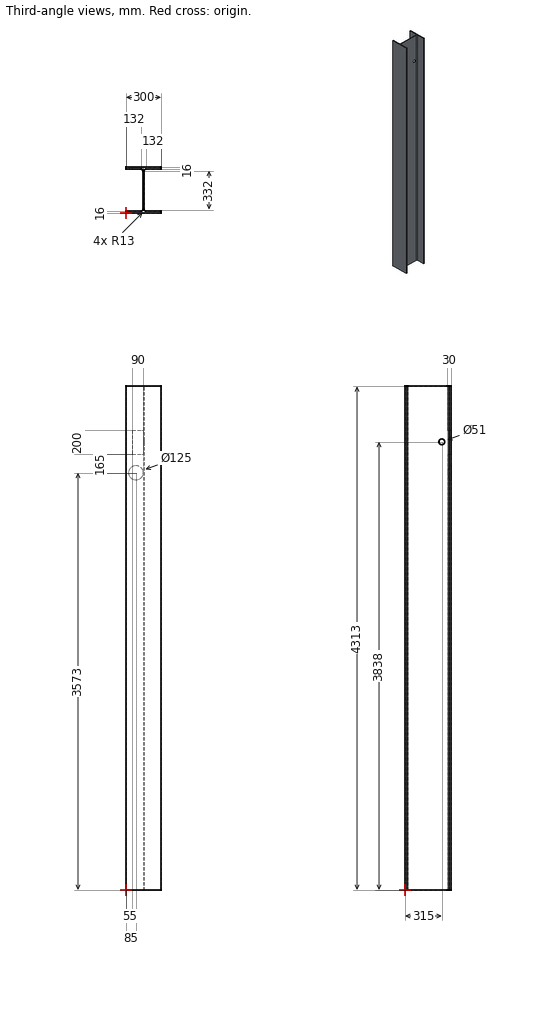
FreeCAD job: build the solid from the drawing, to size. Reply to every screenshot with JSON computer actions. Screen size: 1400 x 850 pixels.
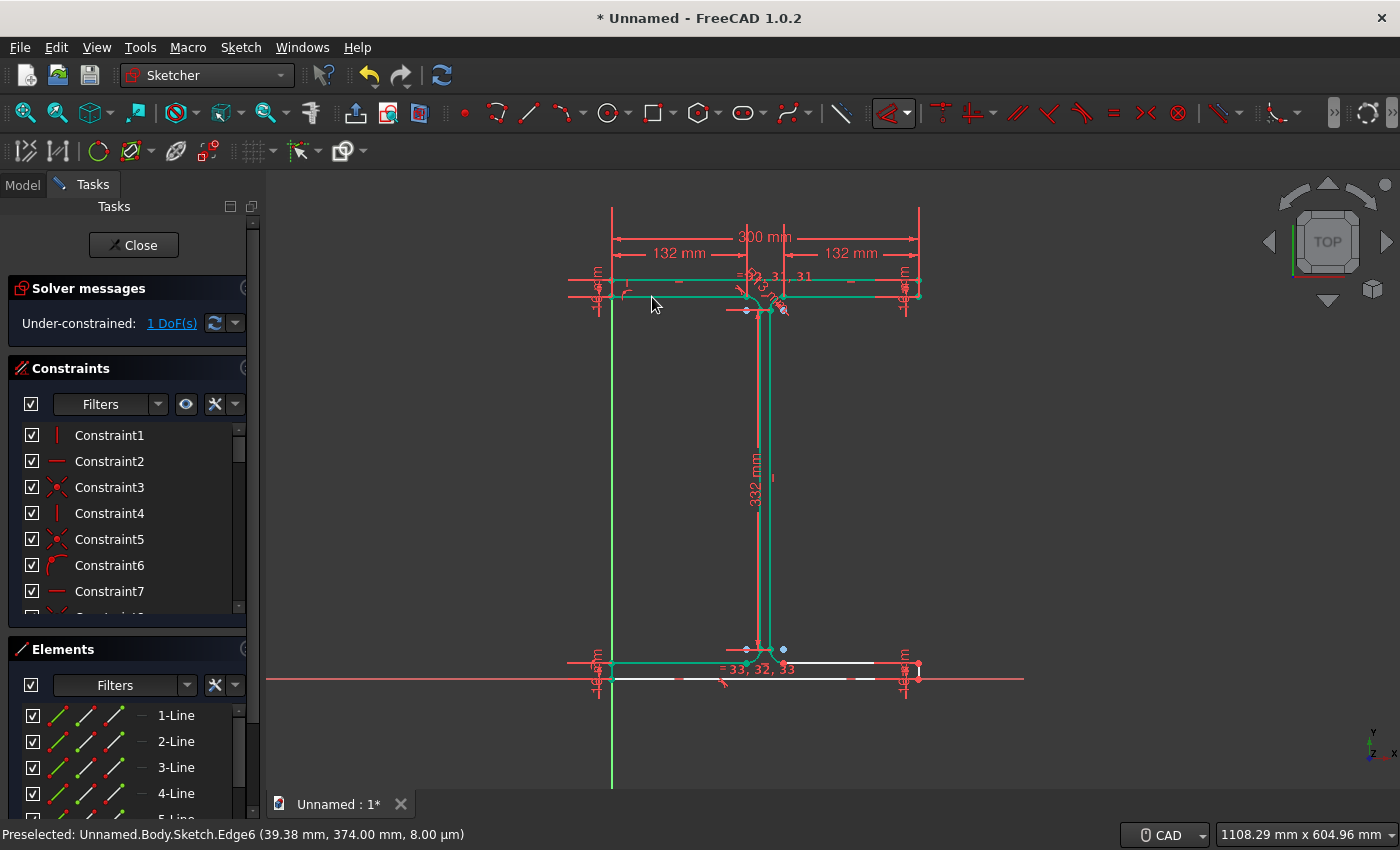
{"action": "left_click", "coordinate": [704, 679]}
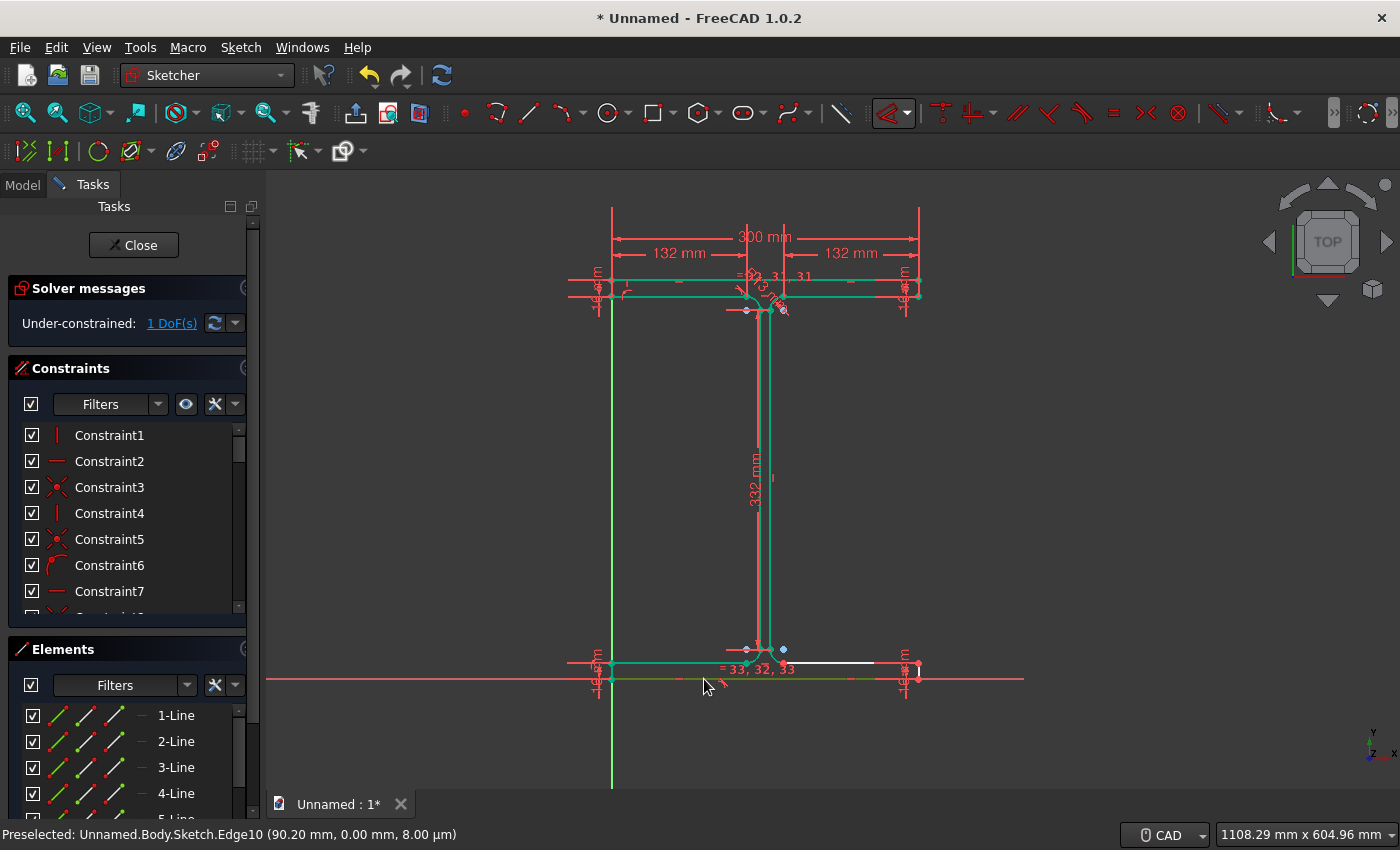
{"action": "key", "text": "l"}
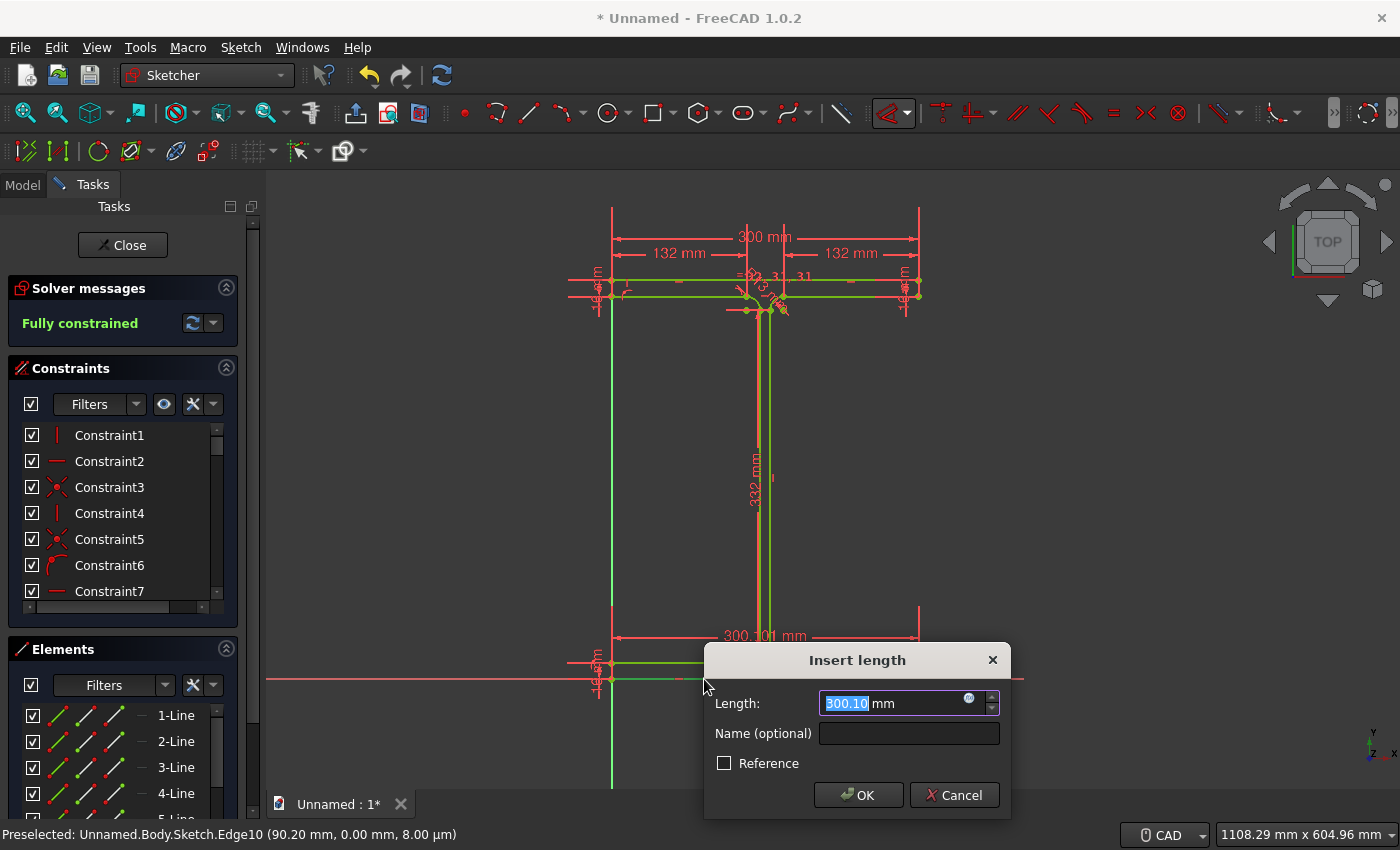
{"action": "type", "text": "300"}
{"action": "key", "text": "Return"}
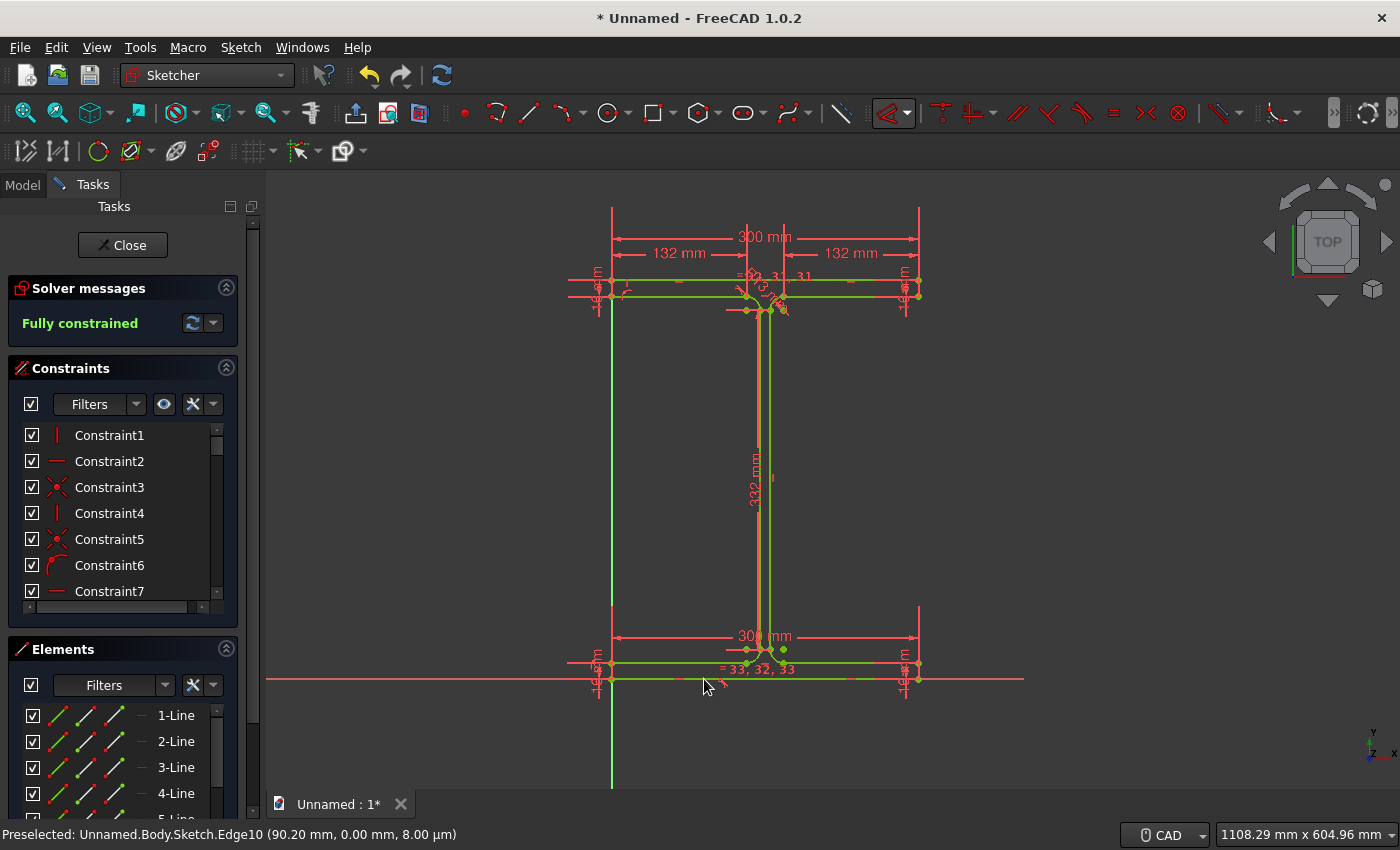
{"action": "left_click", "coordinate": [123, 245]}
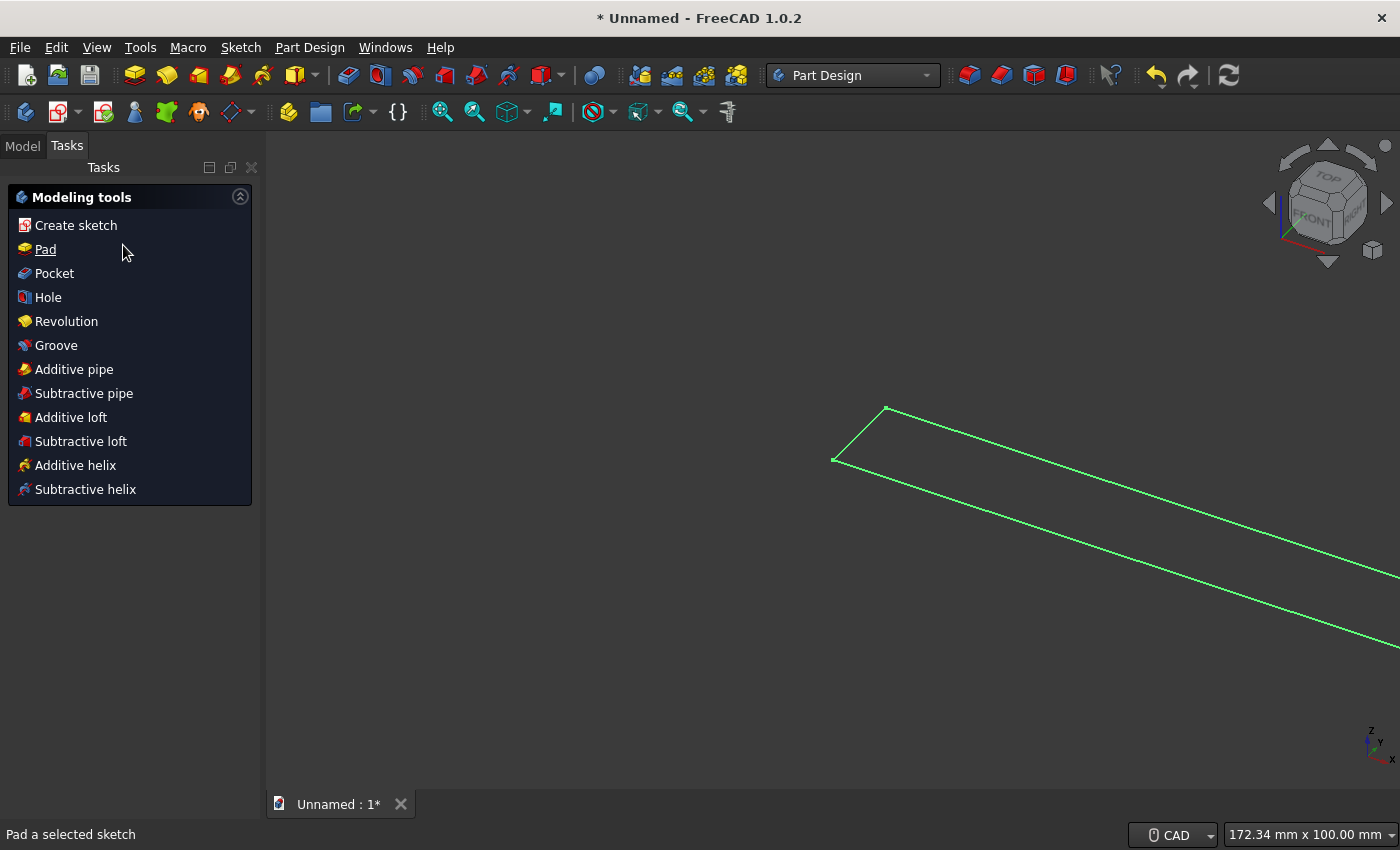
{"action": "left_click", "coordinate": [136, 76]}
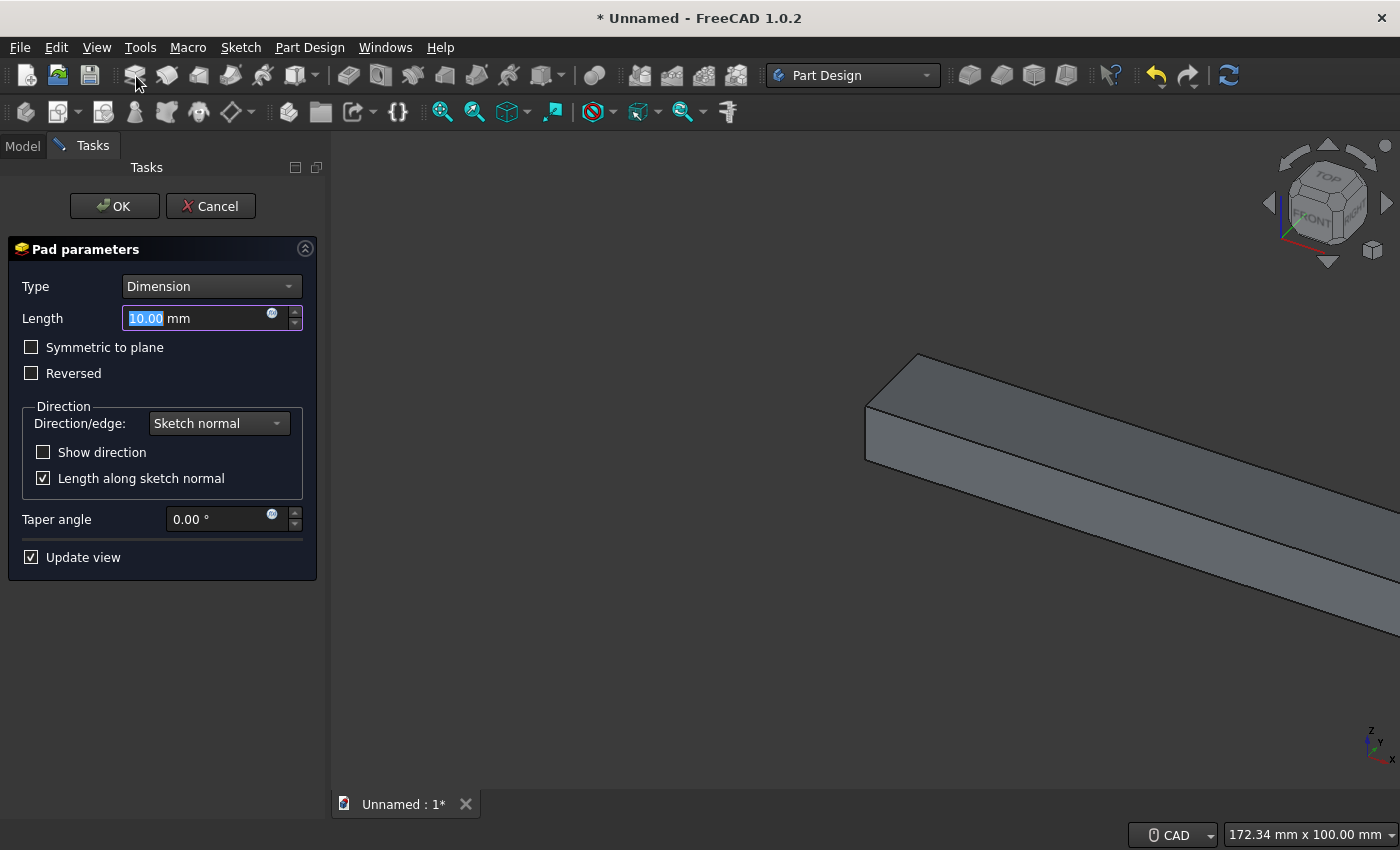
{"action": "type", "text": "4313"}
{"action": "key", "text": "Tab"}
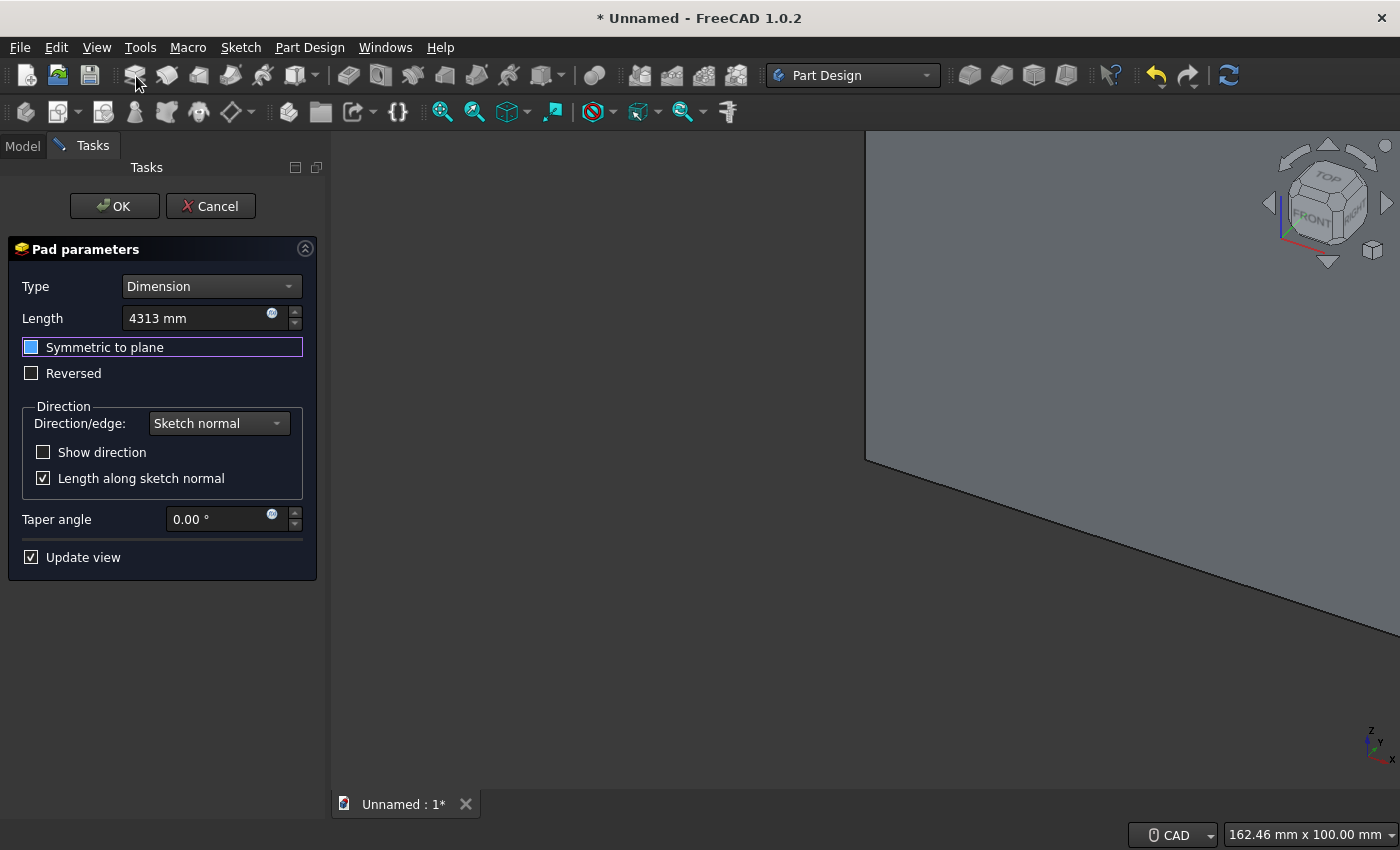
{"action": "left_click", "coordinate": [115, 206]}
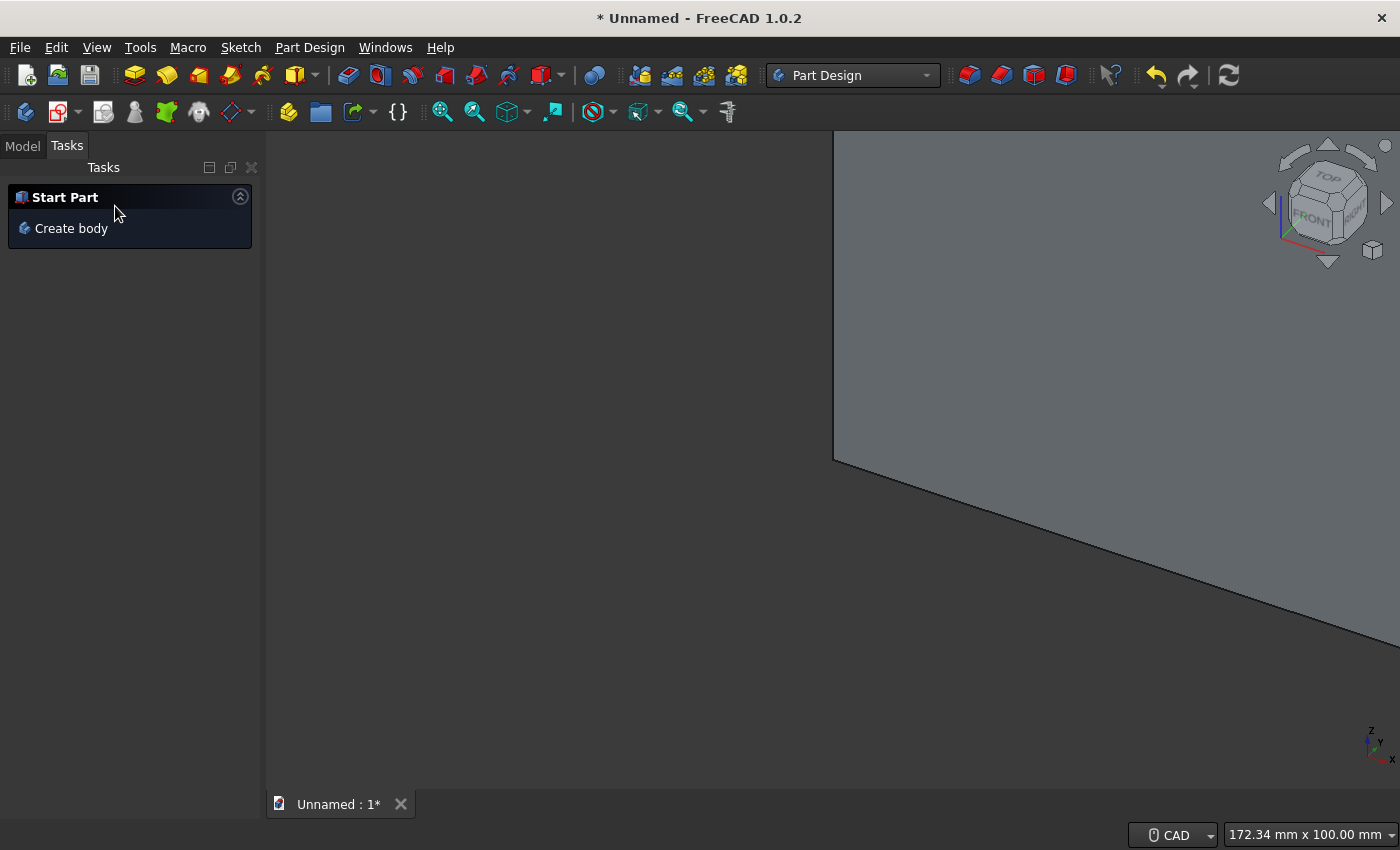
{"action": "left_click", "coordinate": [444, 112]}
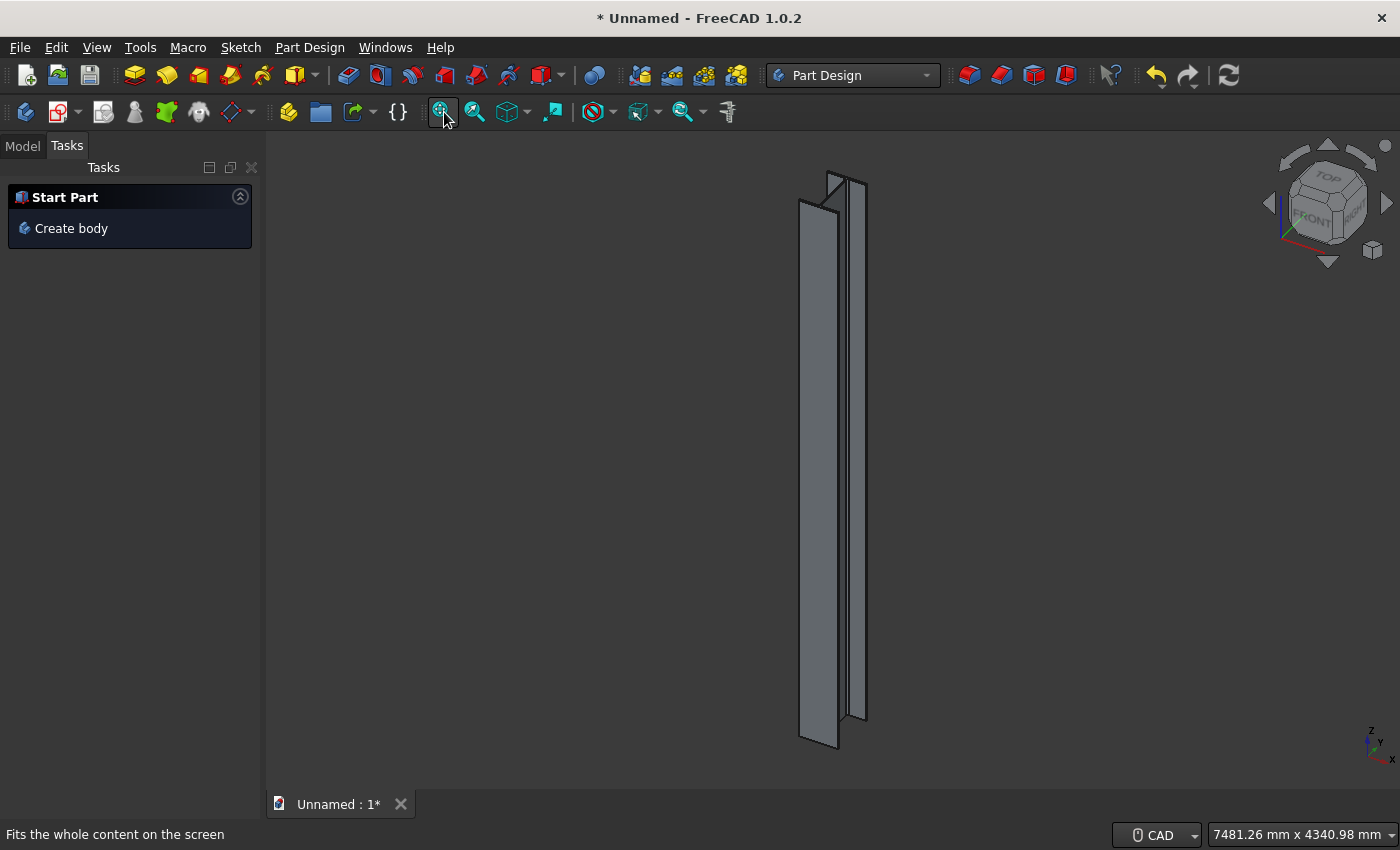
{"action": "key", "text": "4"}